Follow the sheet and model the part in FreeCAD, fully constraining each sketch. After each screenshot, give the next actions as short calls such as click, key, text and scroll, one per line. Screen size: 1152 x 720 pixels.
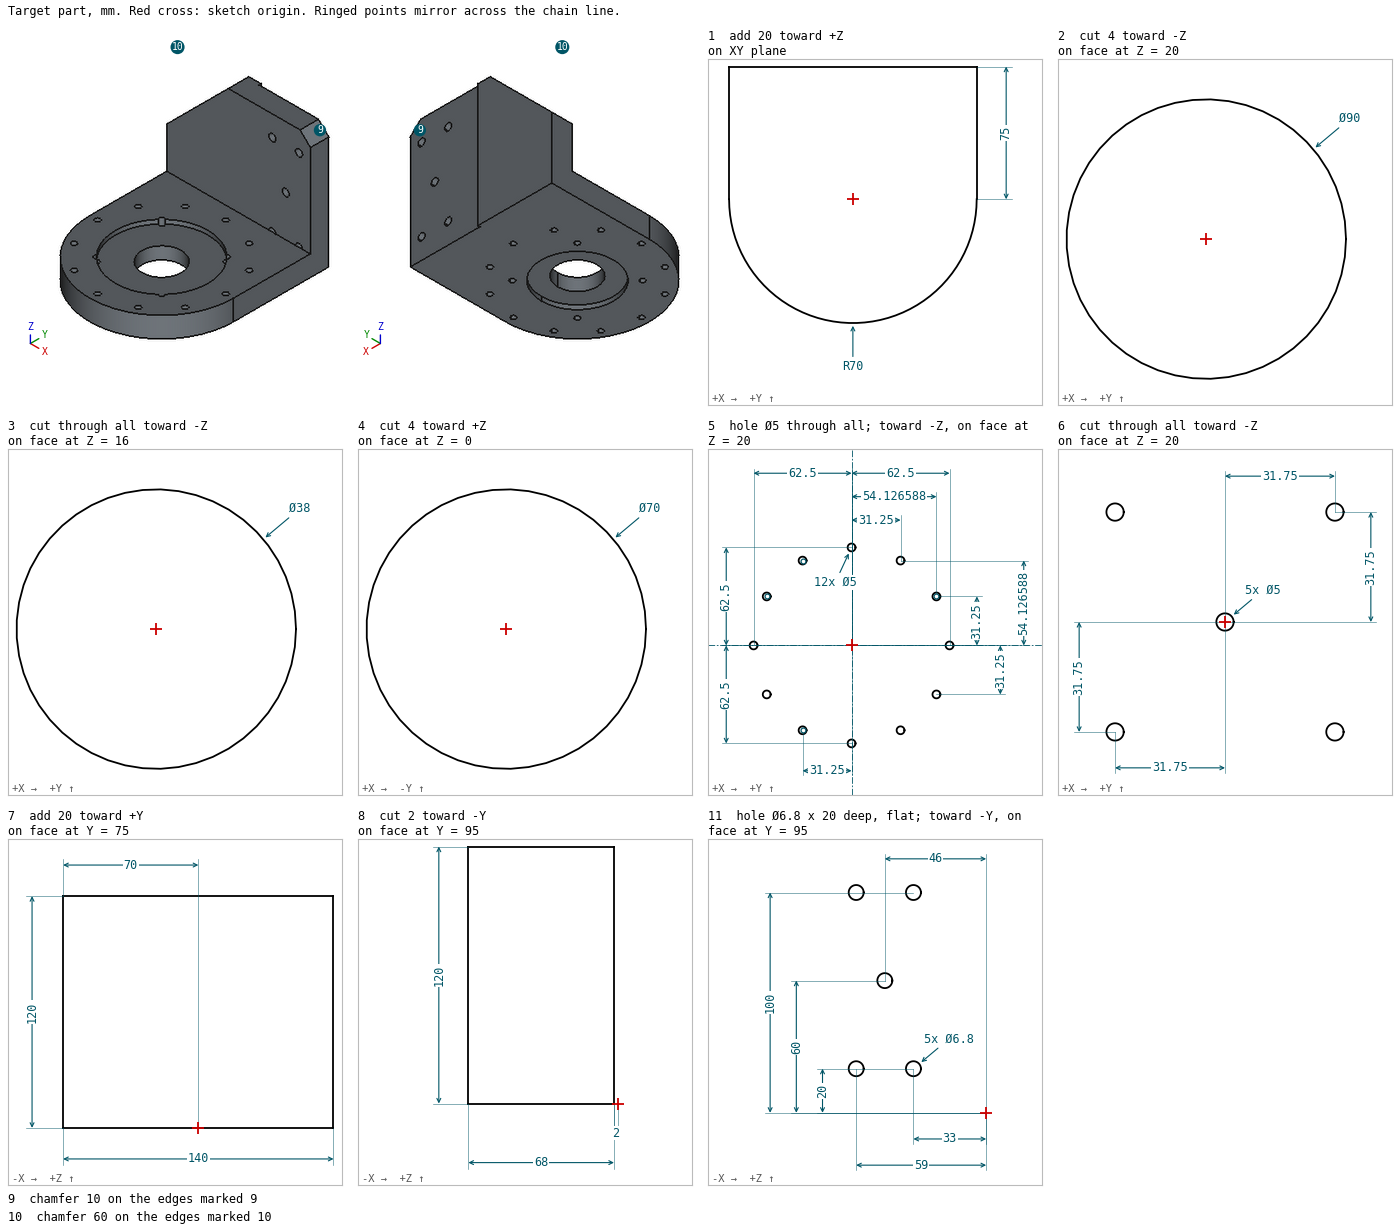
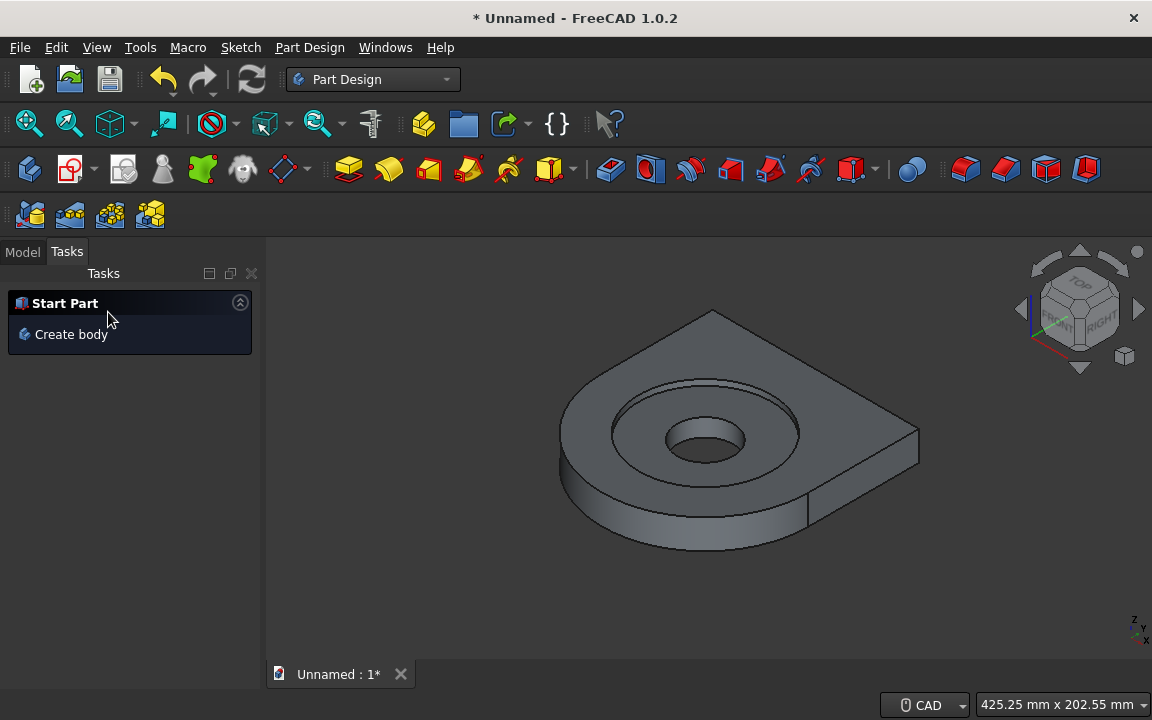
click(711, 361)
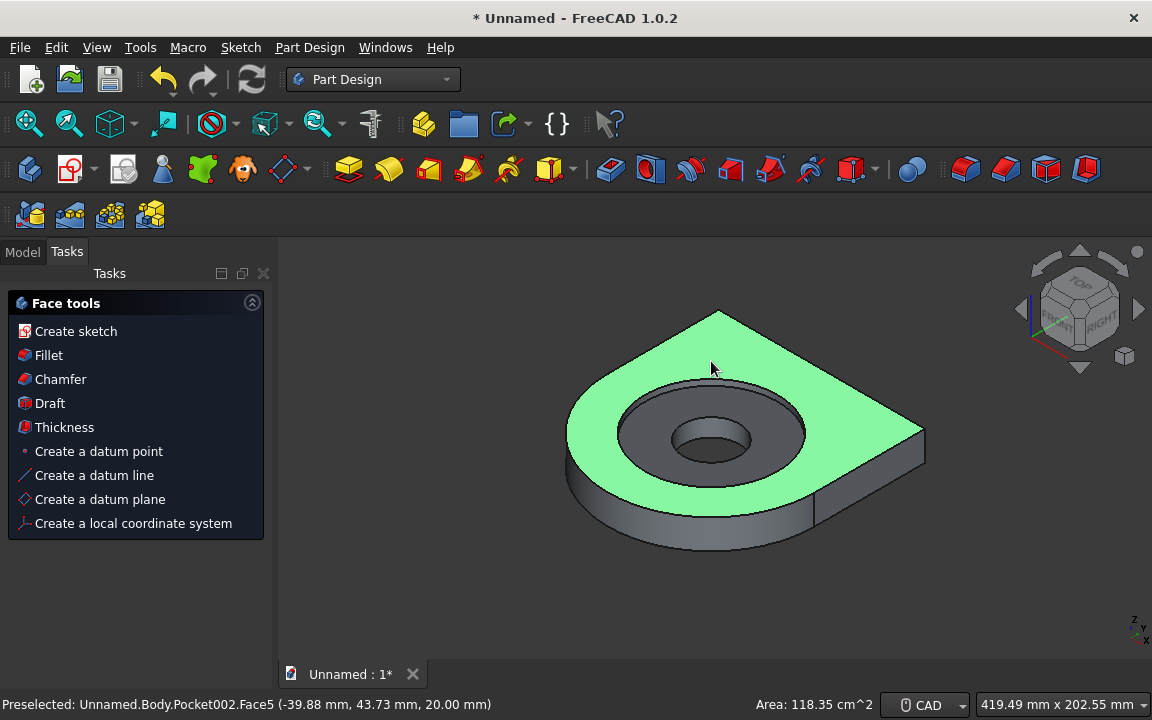
click(70, 170)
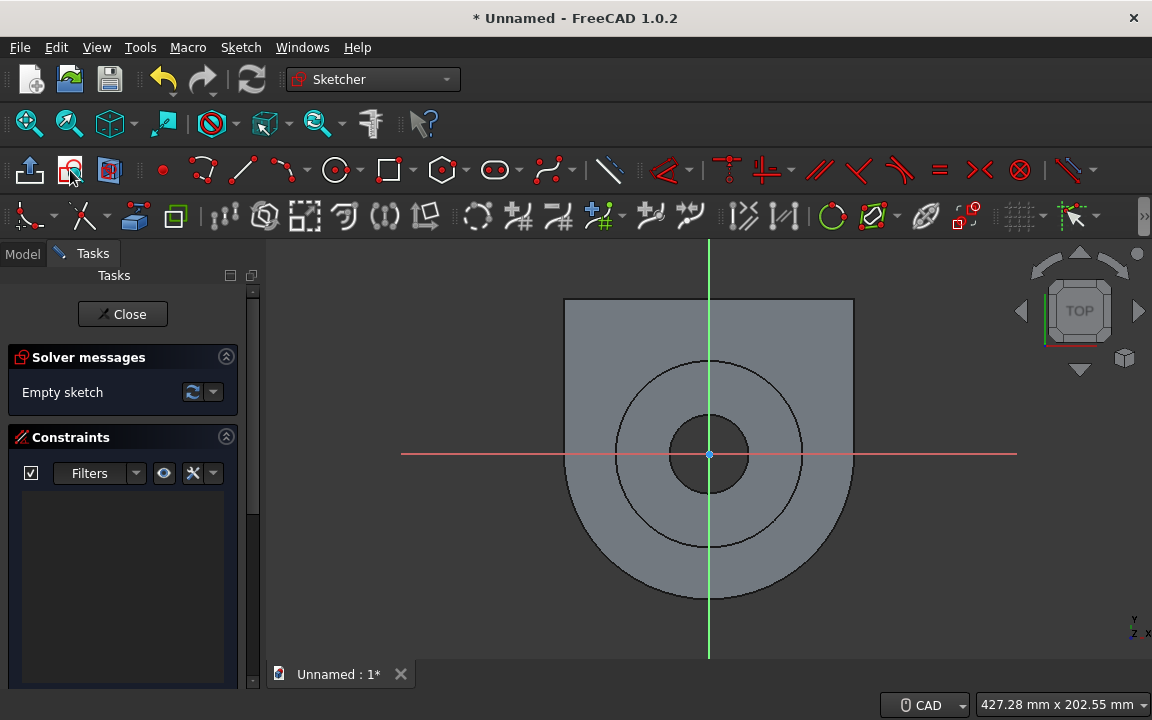
key(g)
key(c)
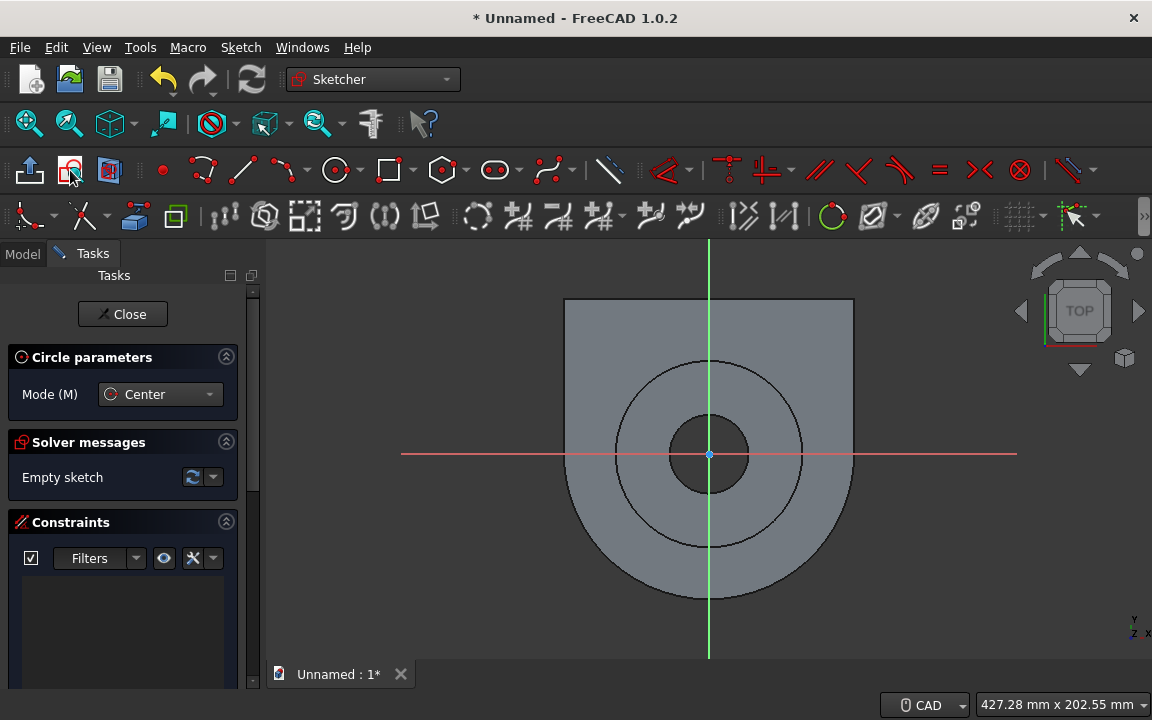
scroll(709, 325, up, 8)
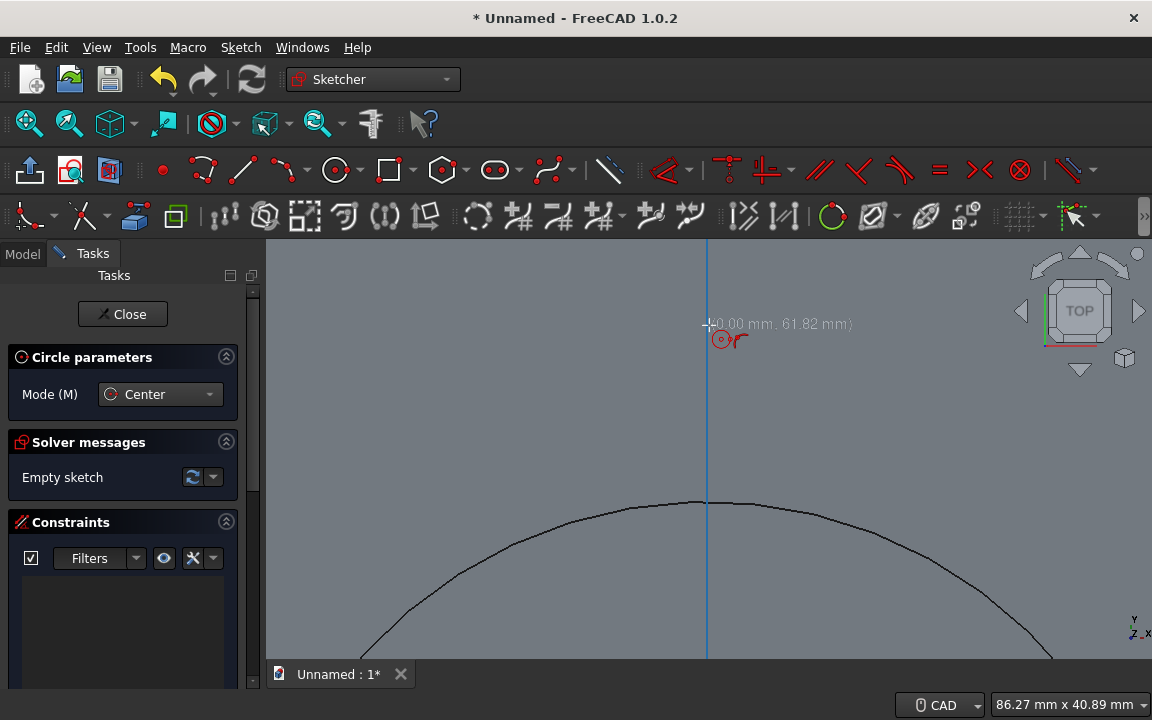
scroll(624, 319, down, 8)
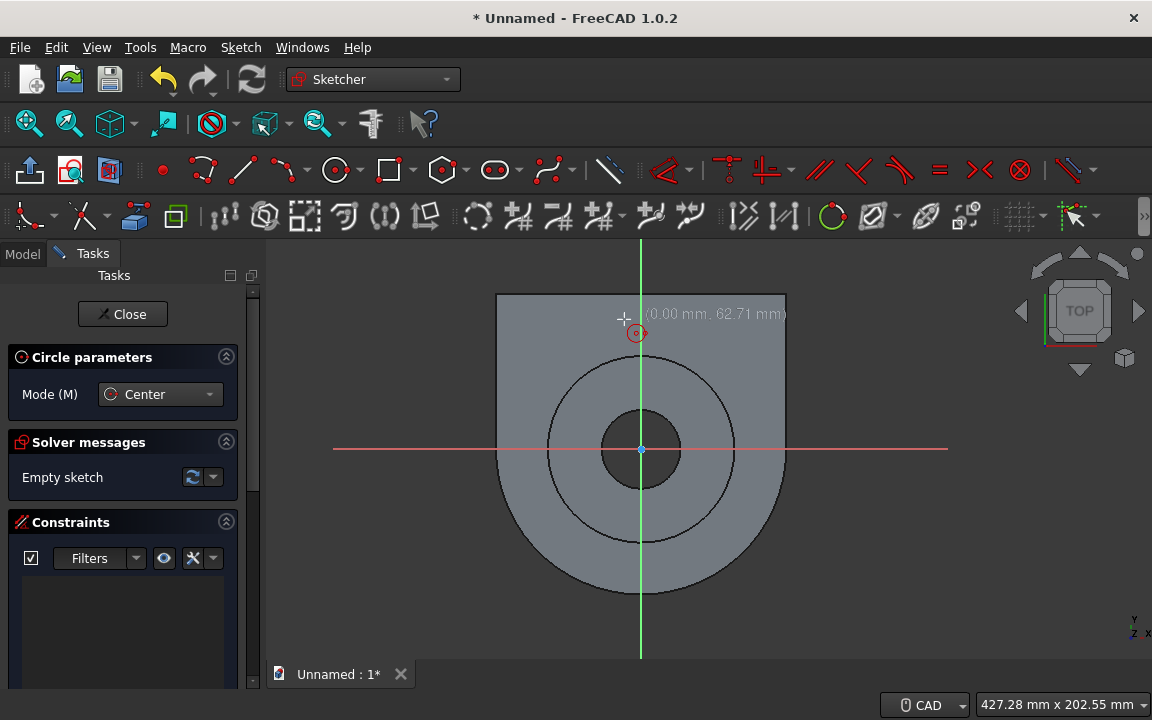
click(641, 320)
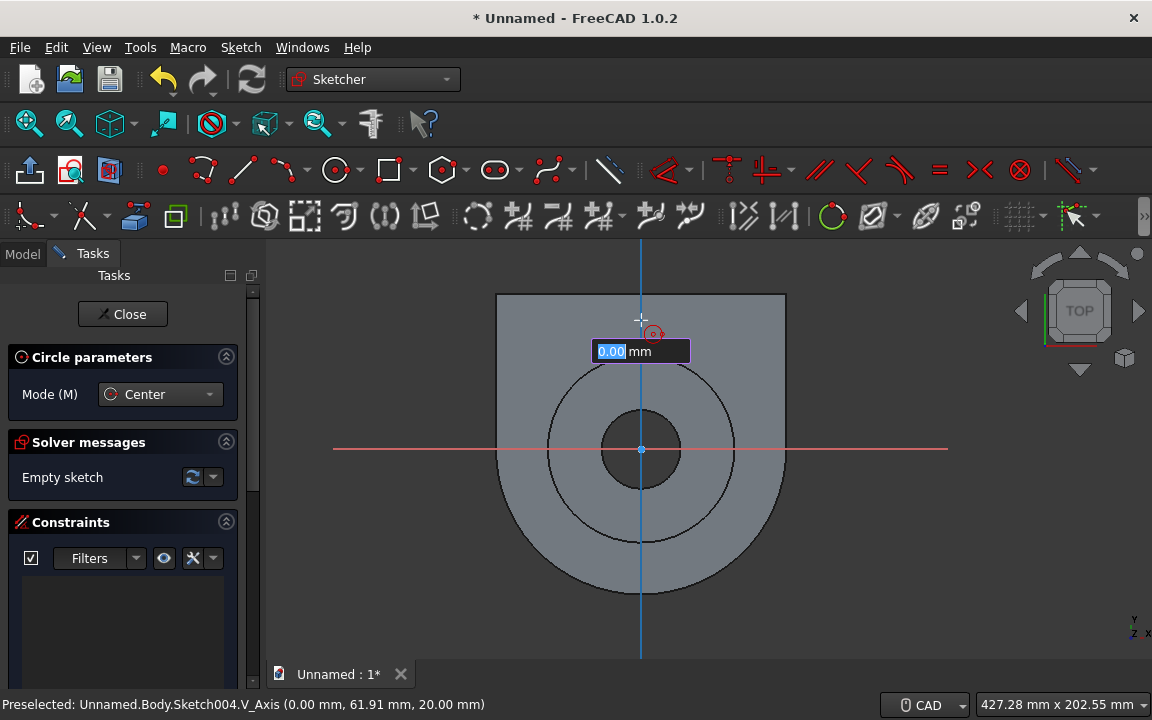
scroll(646, 318, up, 6)
move(645, 318)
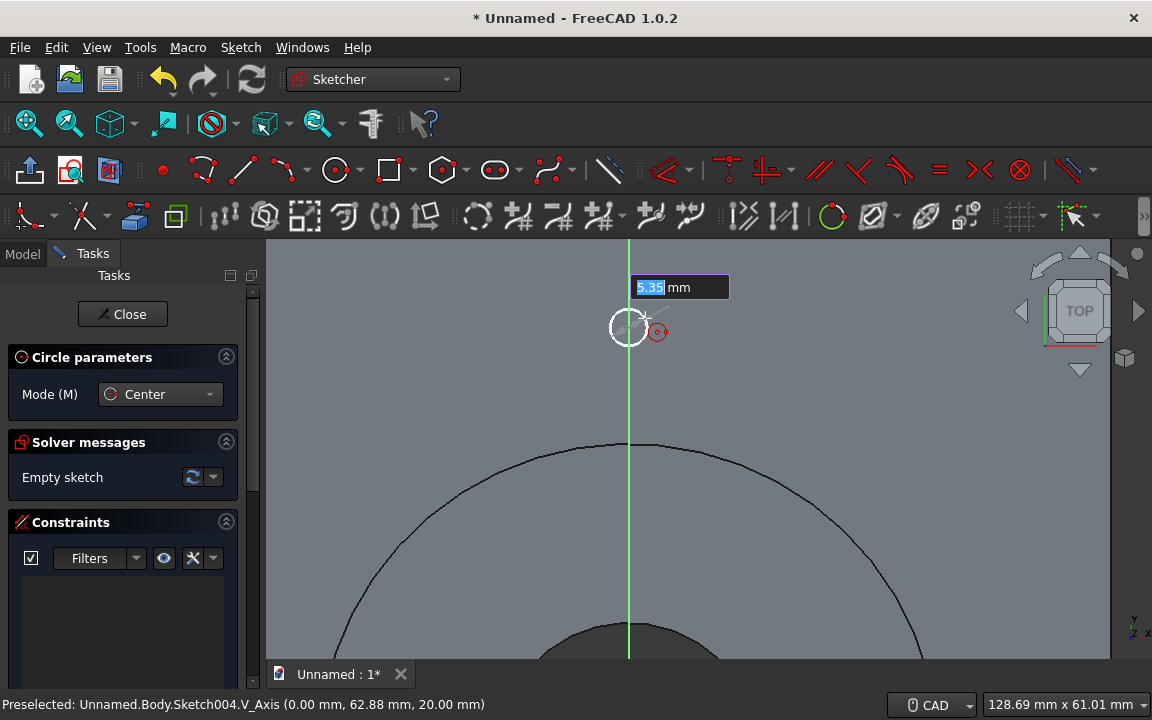
text(5)
key(Return)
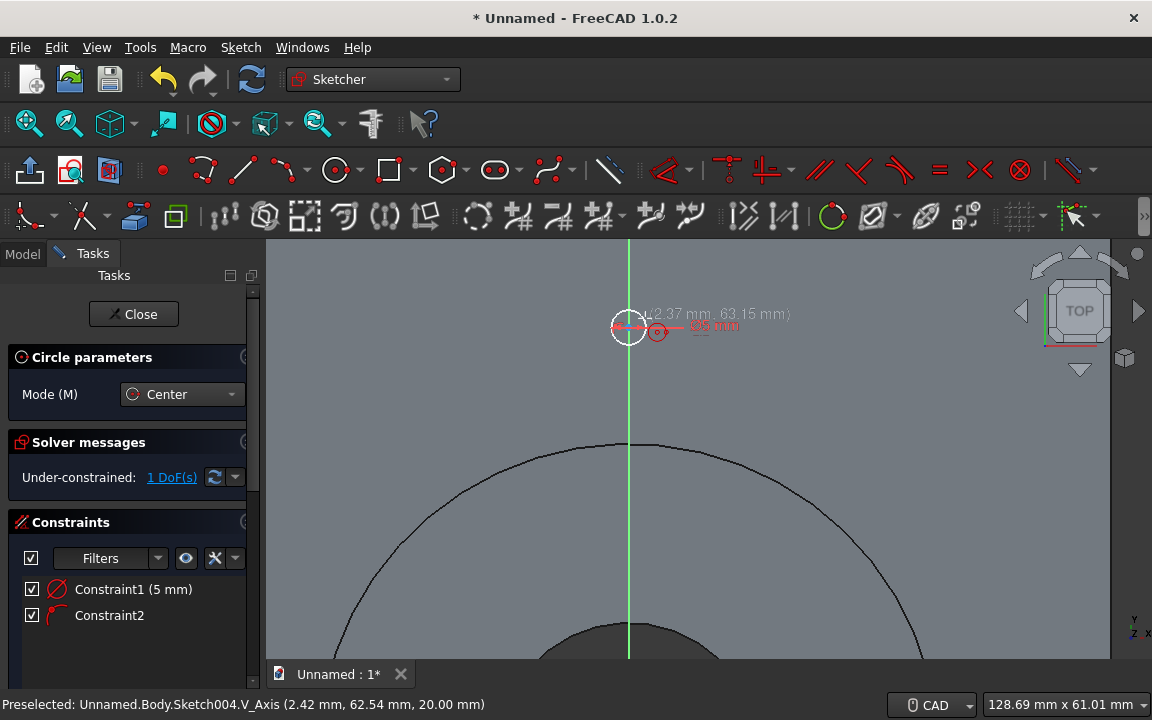
scroll(844, 381, up, 2)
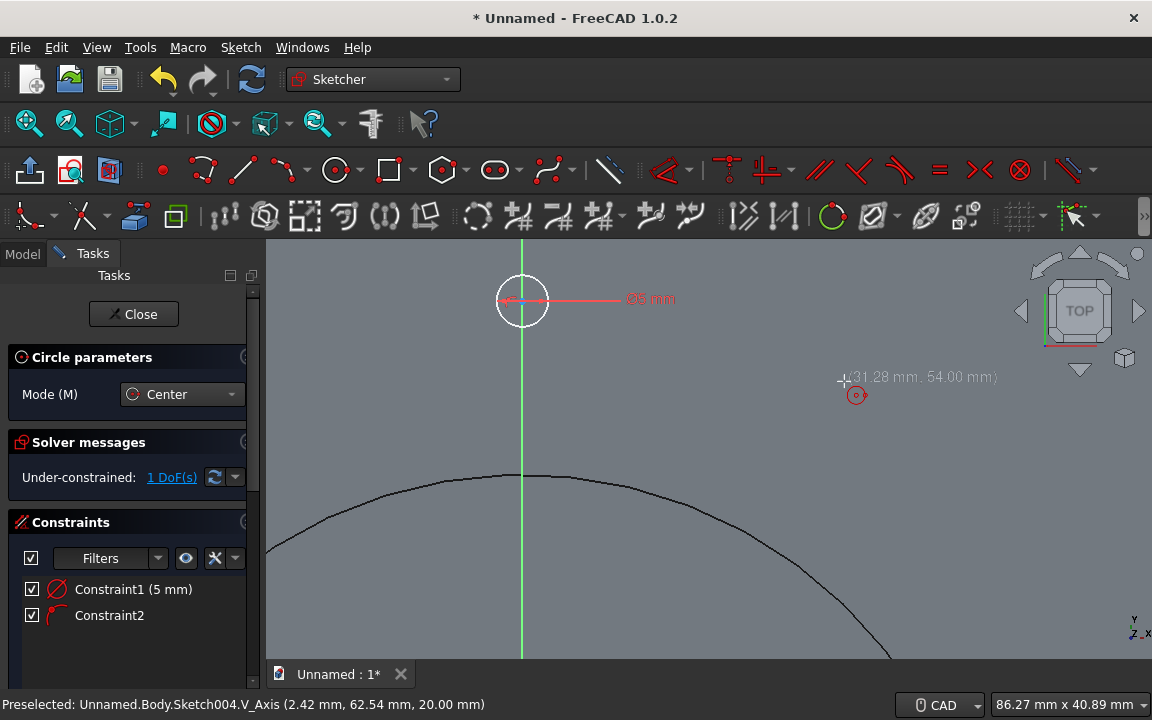
scroll(670, 326, down, 8)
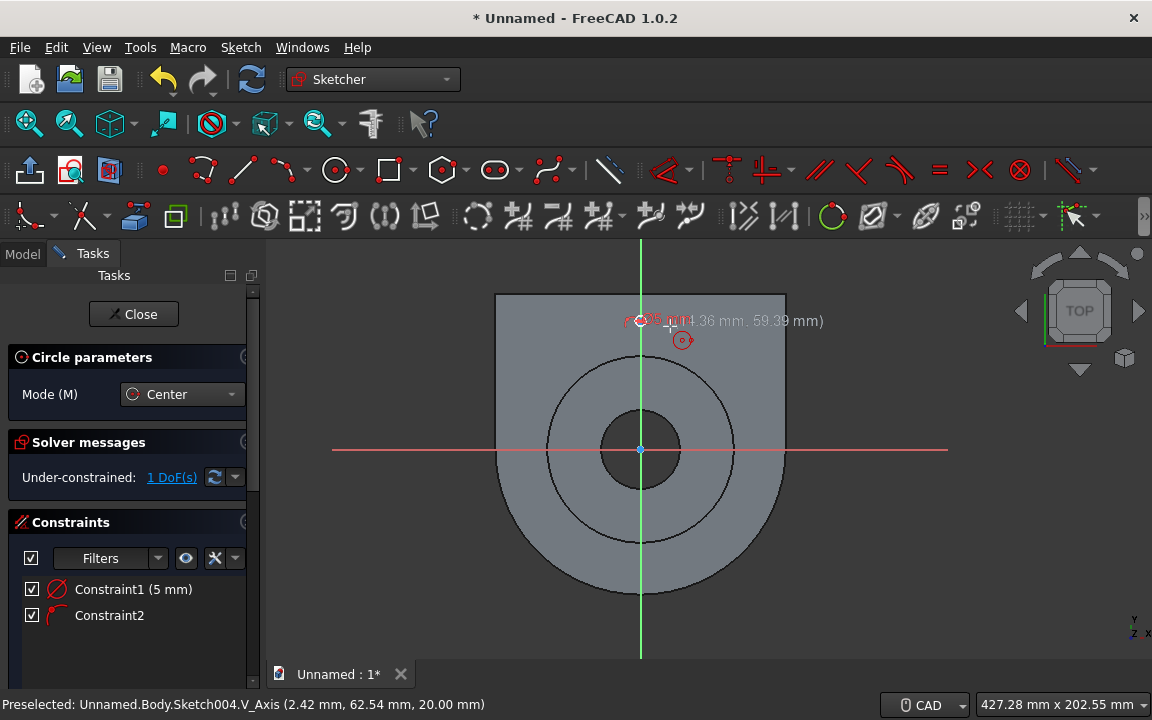
click(705, 337)
move(709, 334)